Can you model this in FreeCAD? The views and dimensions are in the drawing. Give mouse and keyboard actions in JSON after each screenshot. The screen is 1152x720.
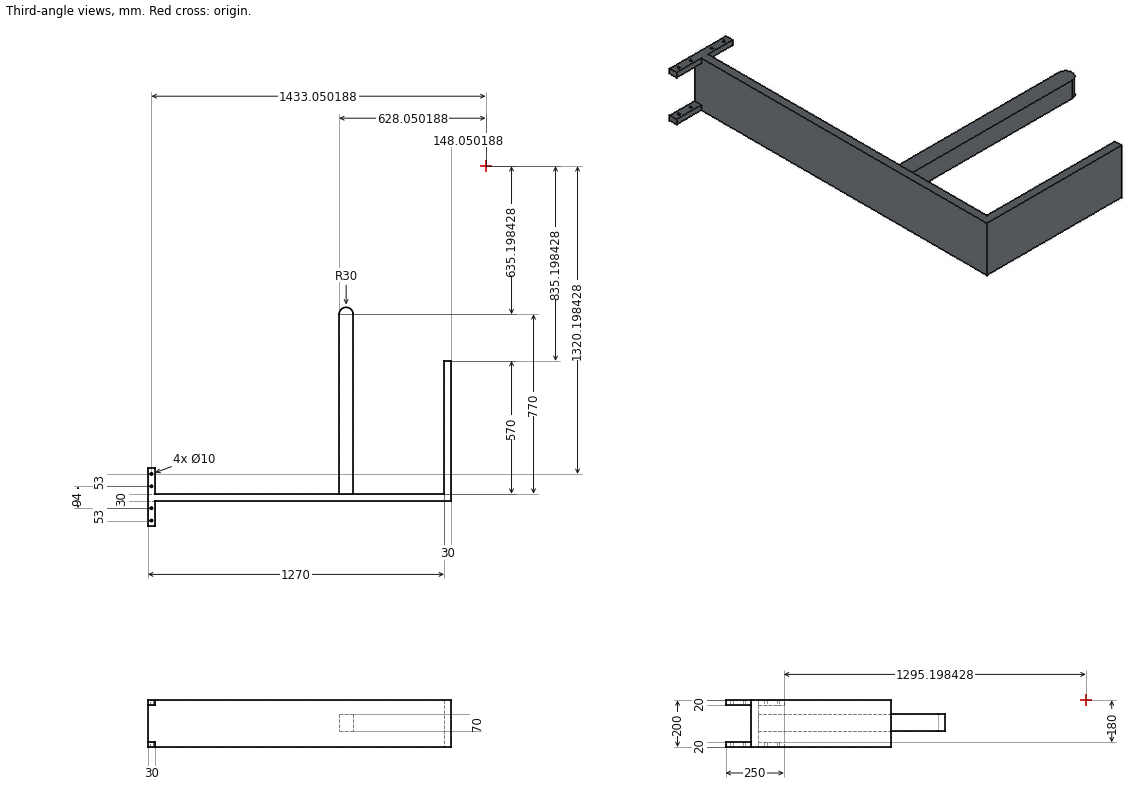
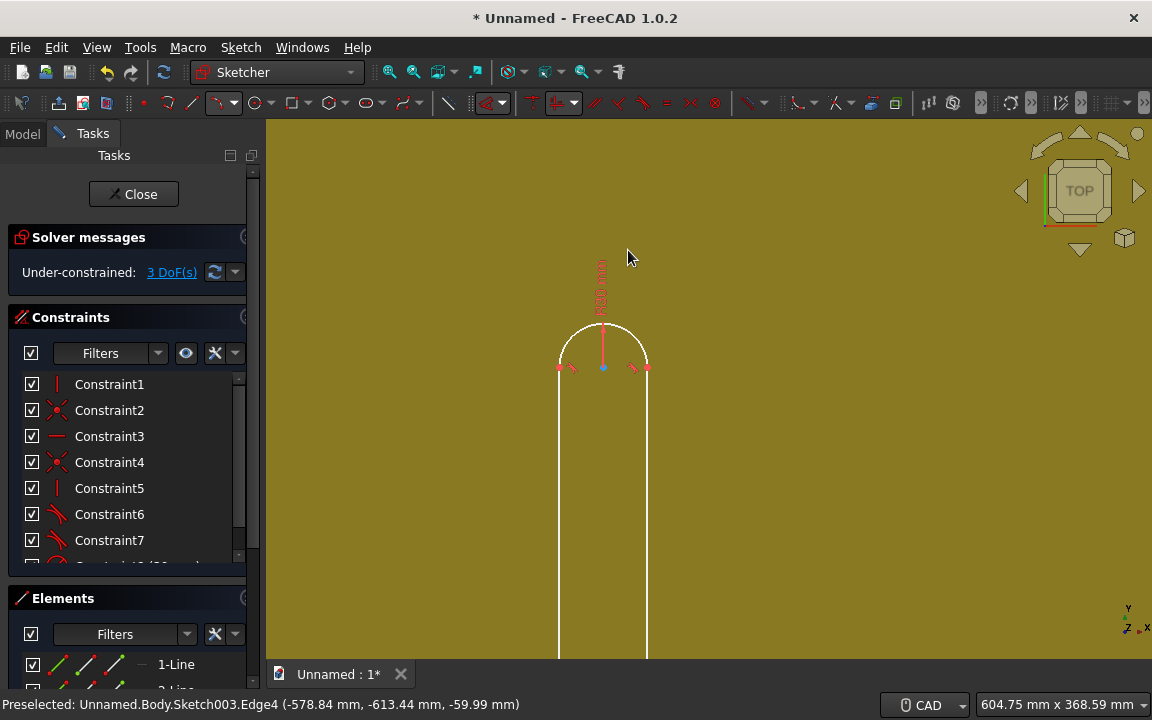
{"action": "scroll", "coordinate": [566, 374], "scroll_direction": "down", "scroll_amount": 9}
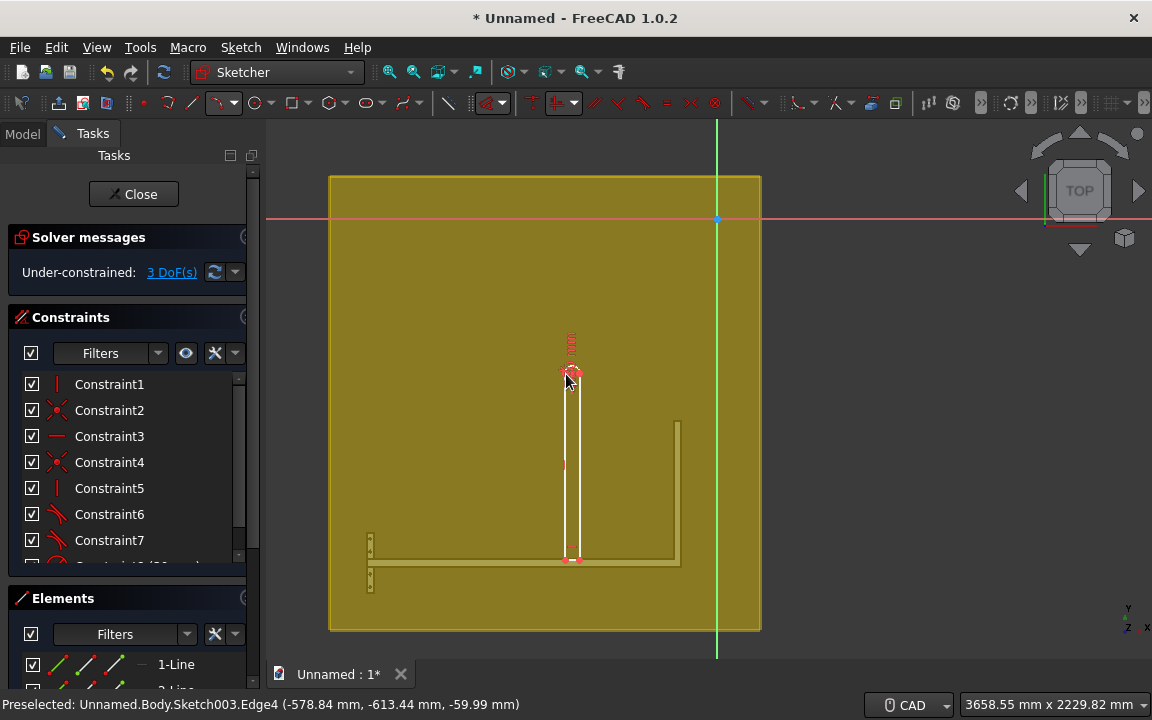
{"action": "left_click", "coordinate": [565, 411]}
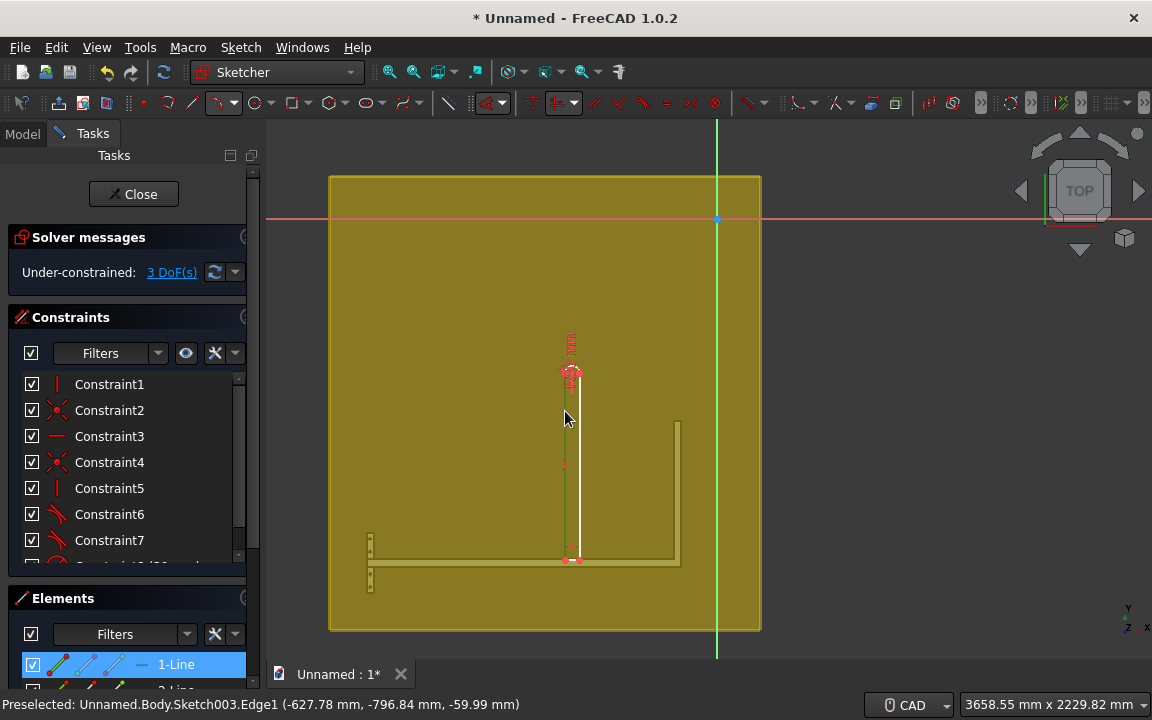
{"action": "left_click", "coordinate": [504, 104]}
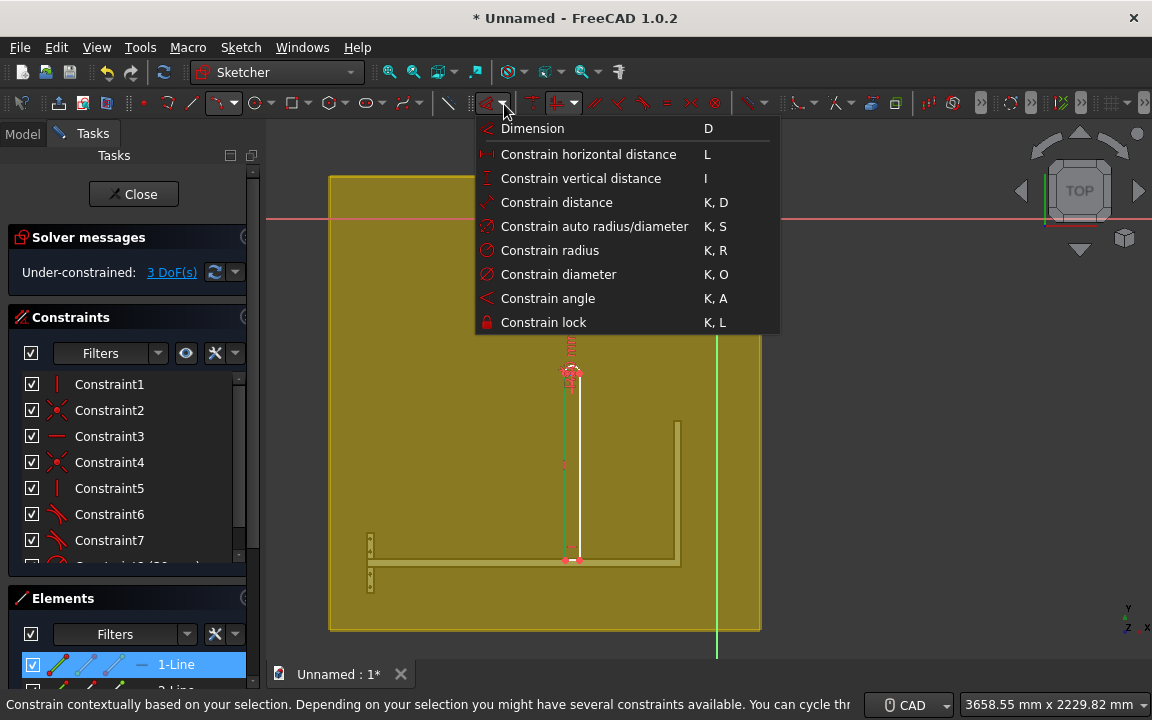
{"action": "left_click", "coordinate": [628, 178]}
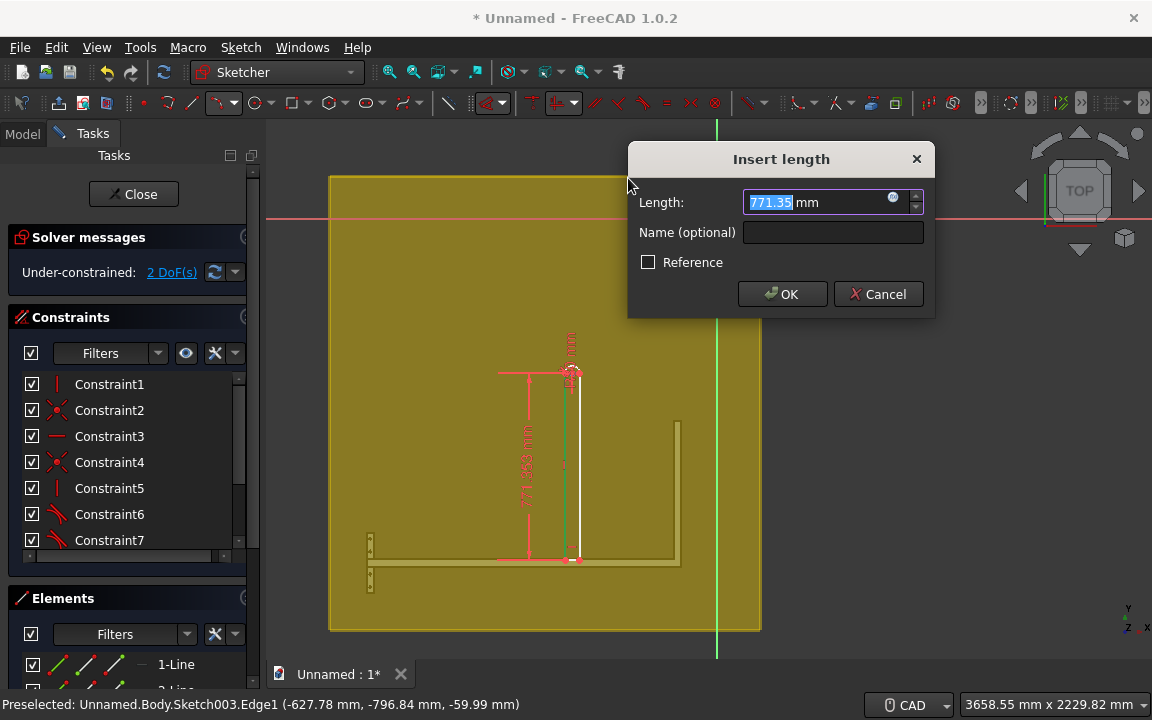
{"action": "type", "text": "770"}
{"action": "key", "text": "Return"}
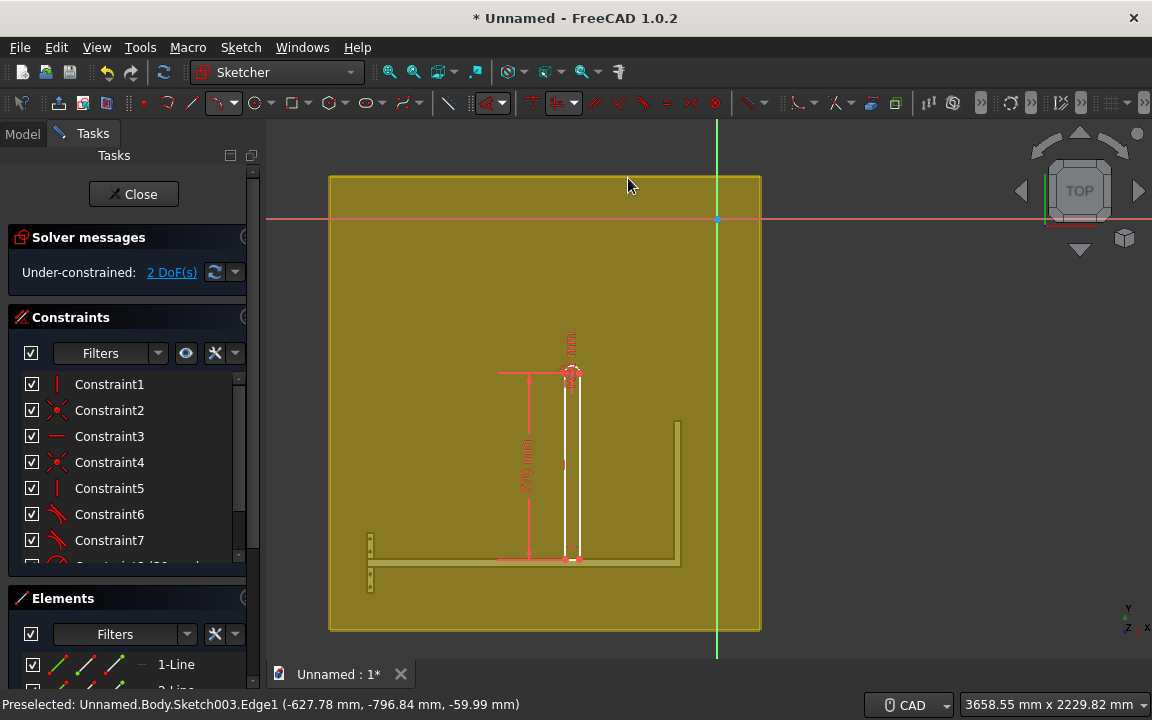
{"action": "scroll", "coordinate": [565, 373], "scroll_direction": "up", "scroll_amount": 3}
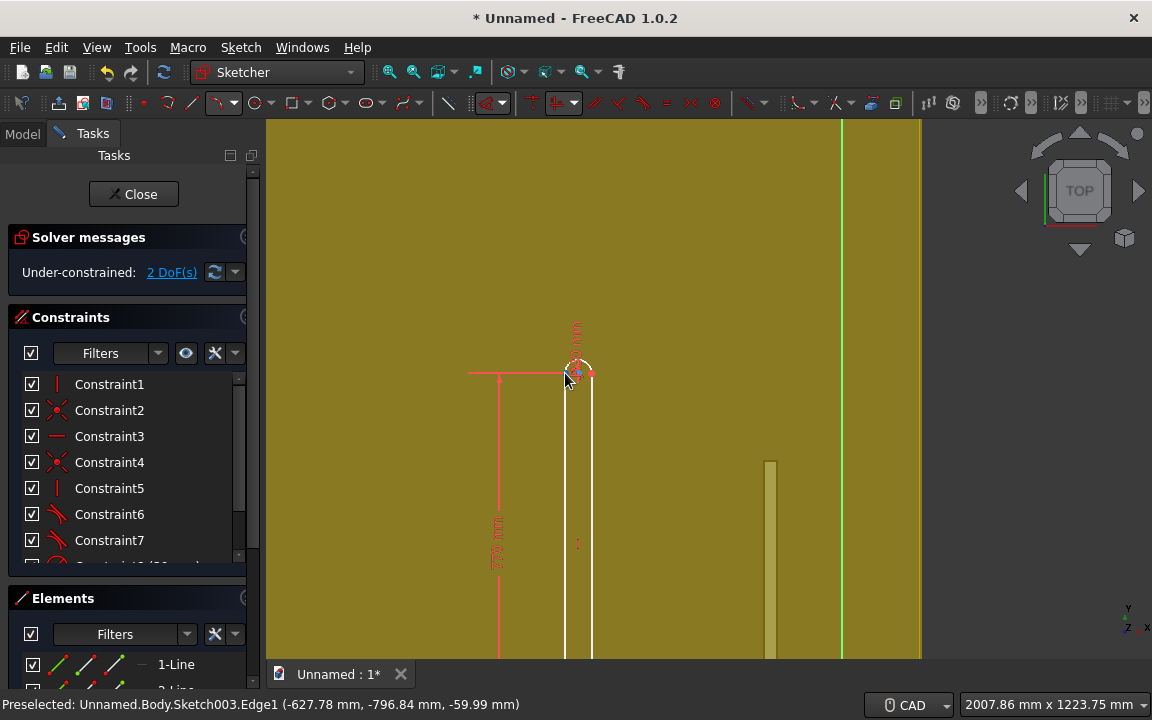
{"action": "left_click", "coordinate": [565, 373]}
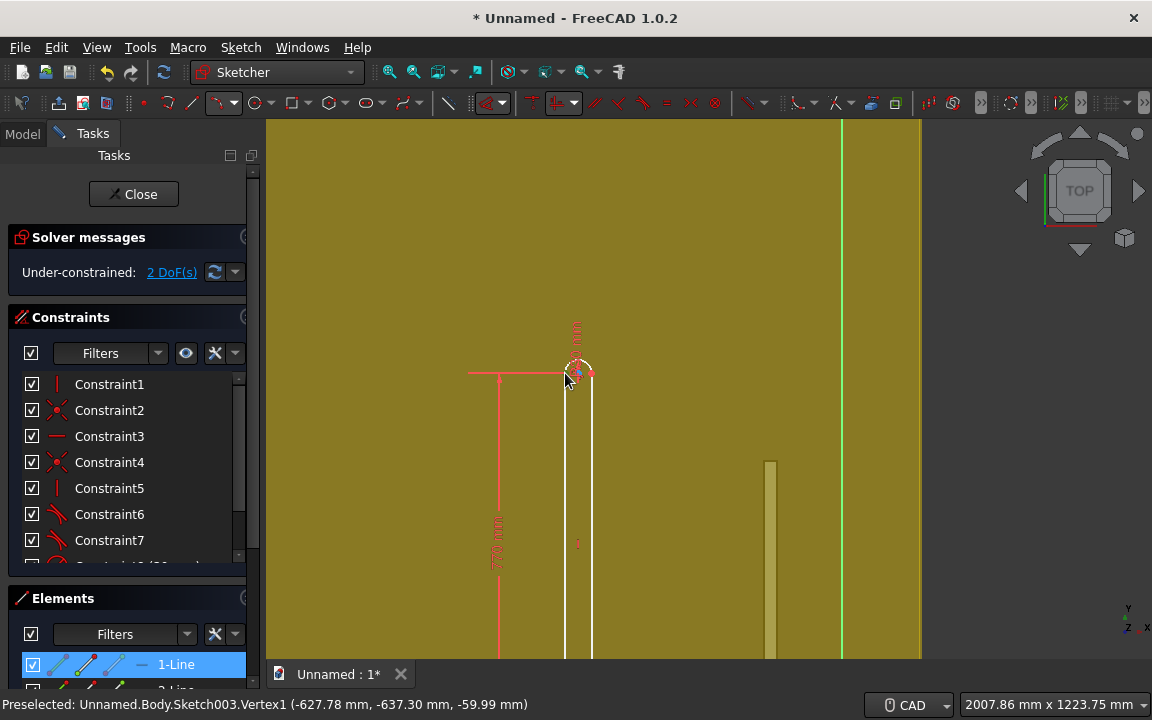
{"action": "key", "text": "l"}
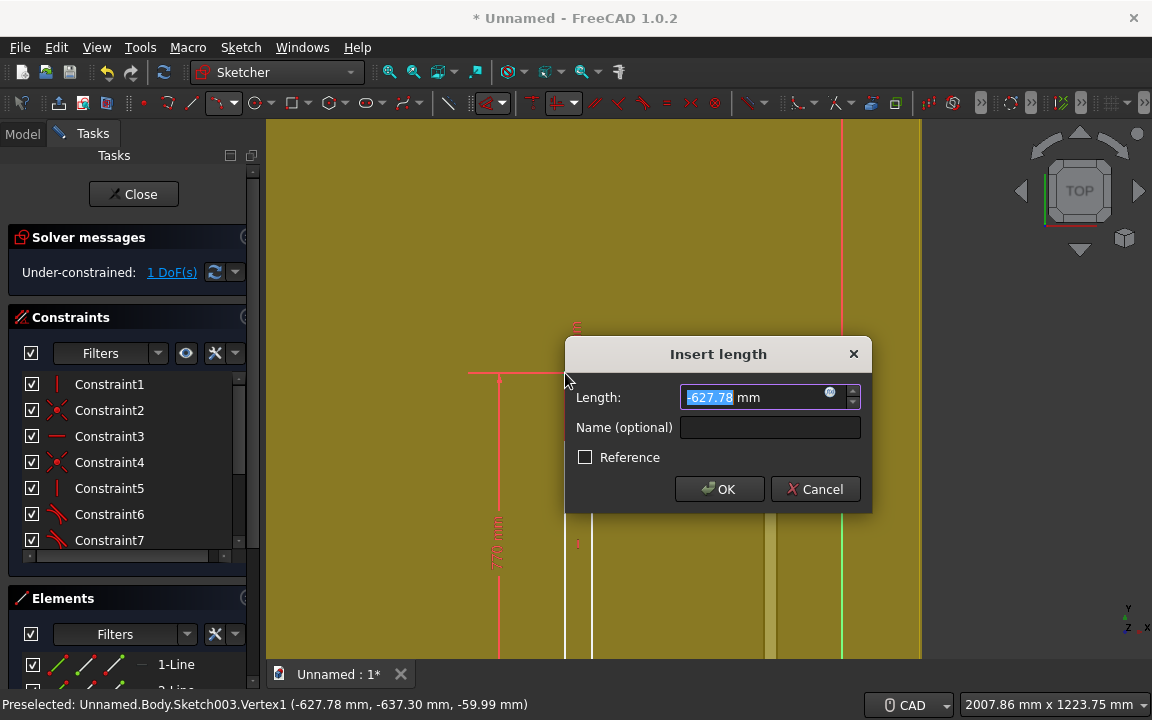
{"action": "type", "text": "-628.050188"}
{"action": "key", "text": "Return"}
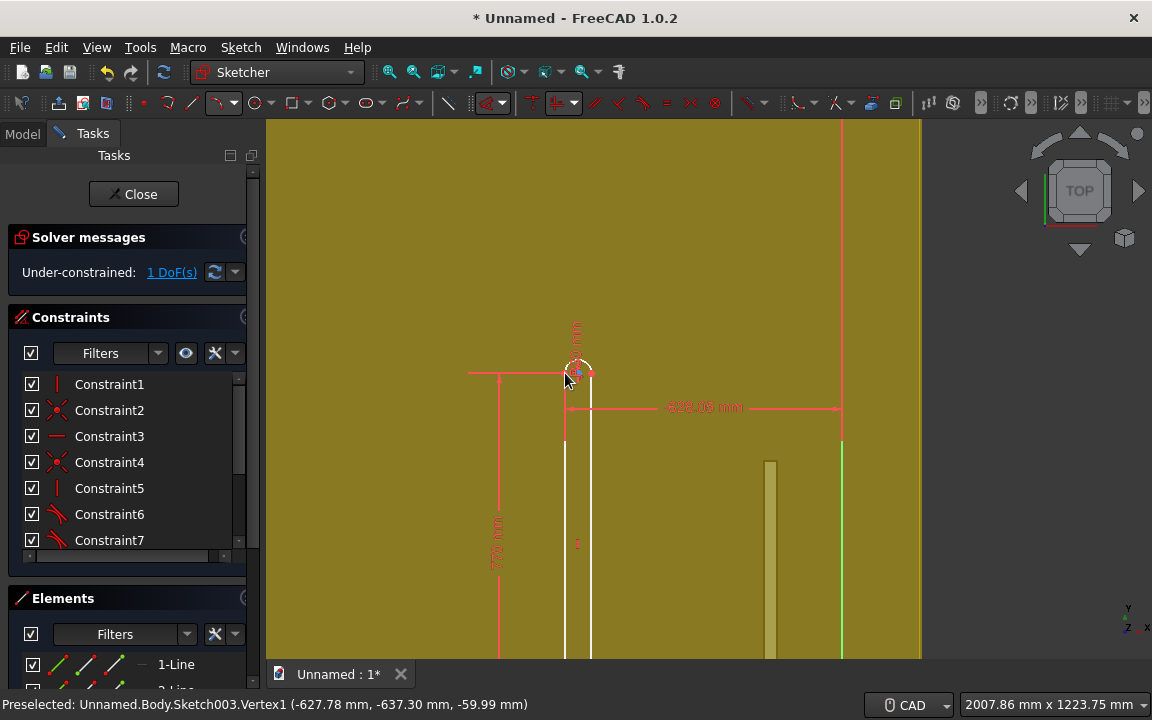
{"action": "left_click", "coordinate": [565, 373]}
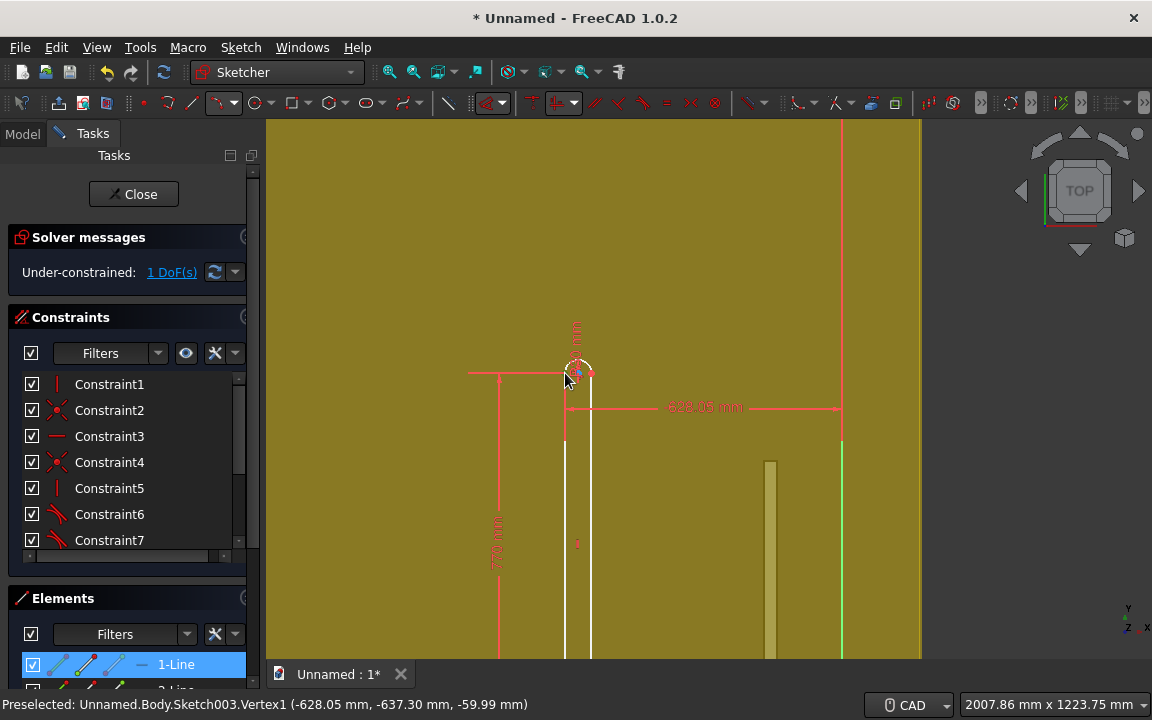
{"action": "left_click", "coordinate": [504, 104]}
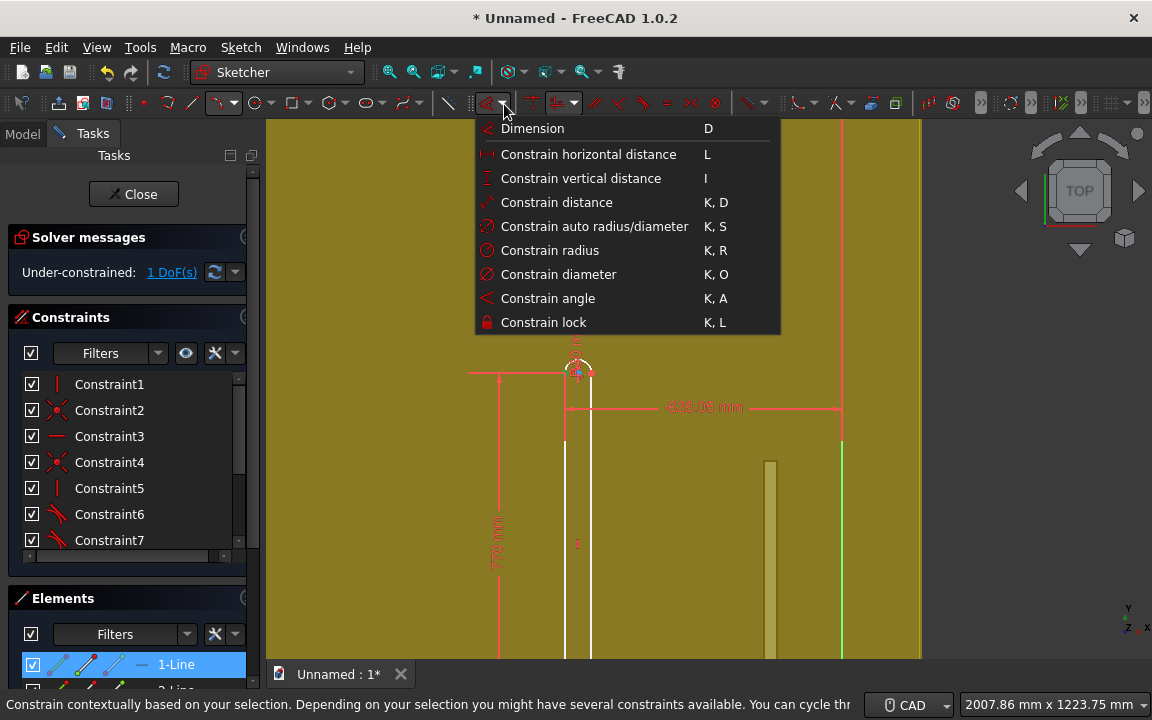
{"action": "left_click", "coordinate": [628, 178]}